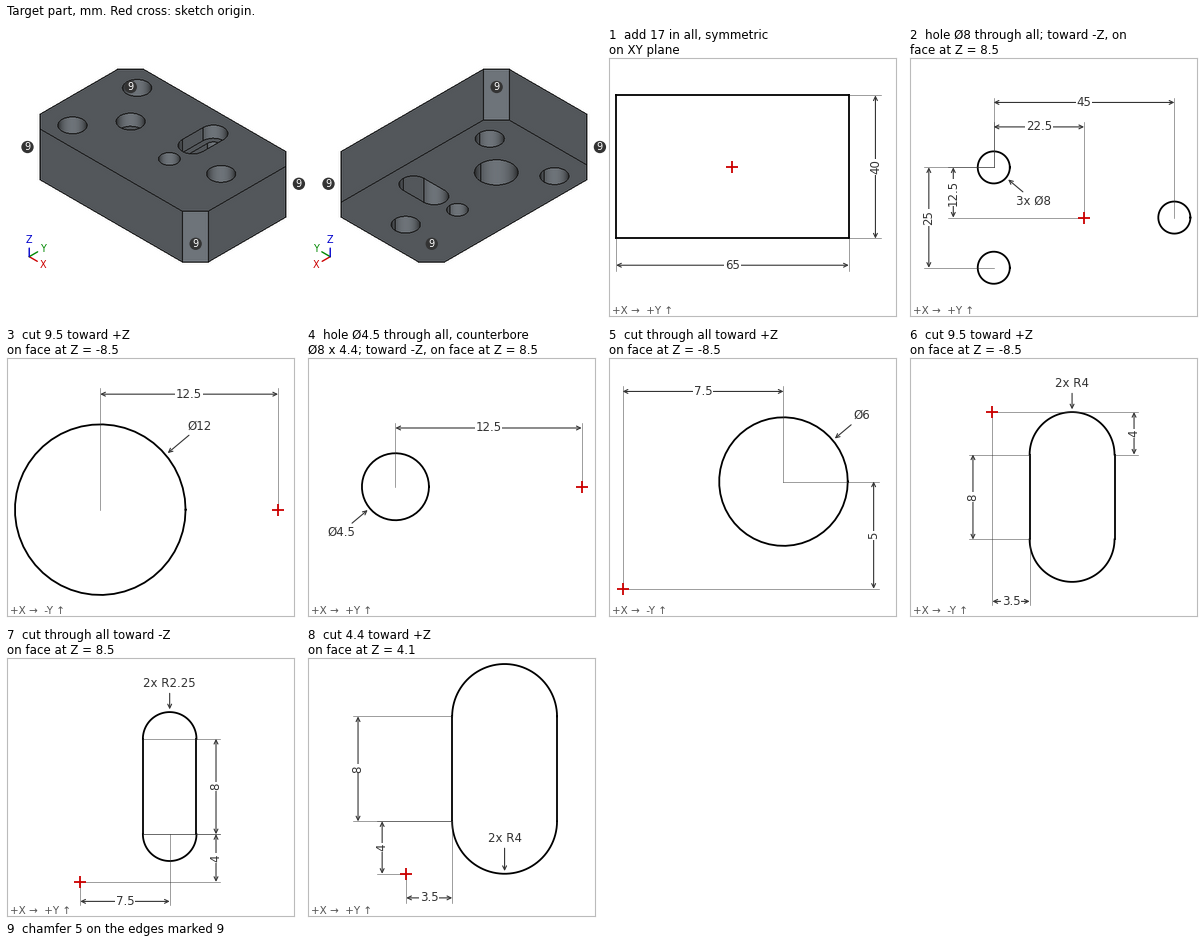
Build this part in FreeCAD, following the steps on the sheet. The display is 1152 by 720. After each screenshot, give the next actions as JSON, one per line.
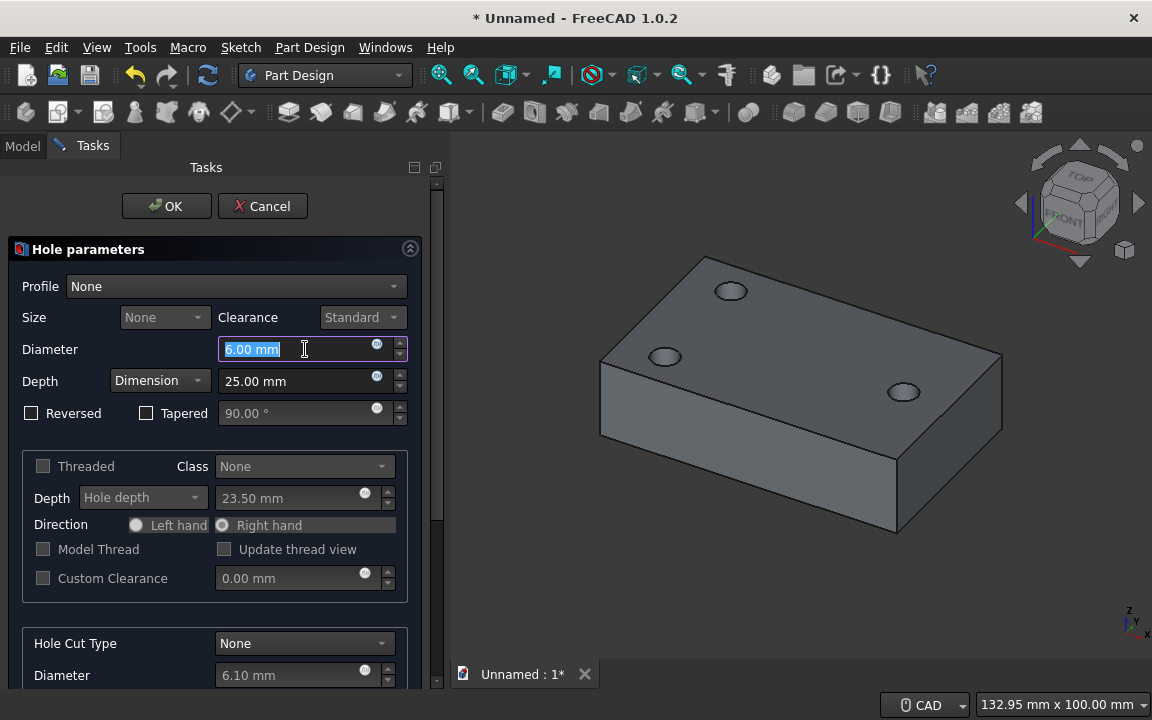
{"action": "type", "text": "8"}
{"action": "key", "text": "Tab"}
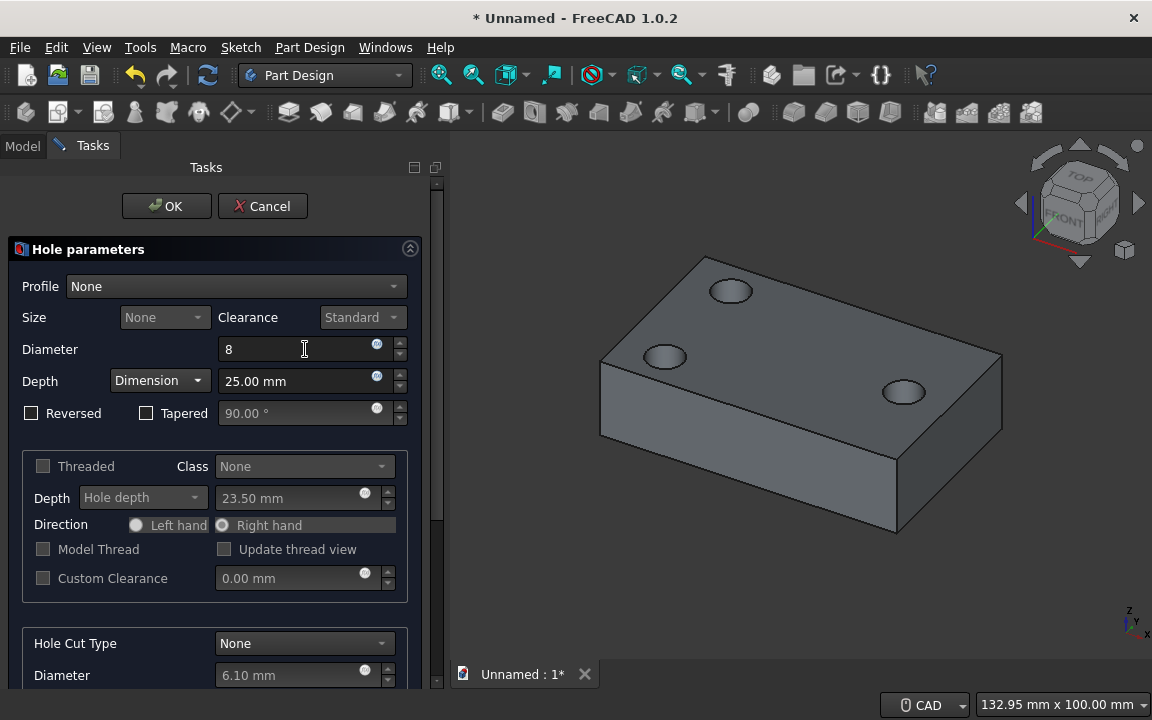
{"action": "left_click", "coordinate": [161, 380]}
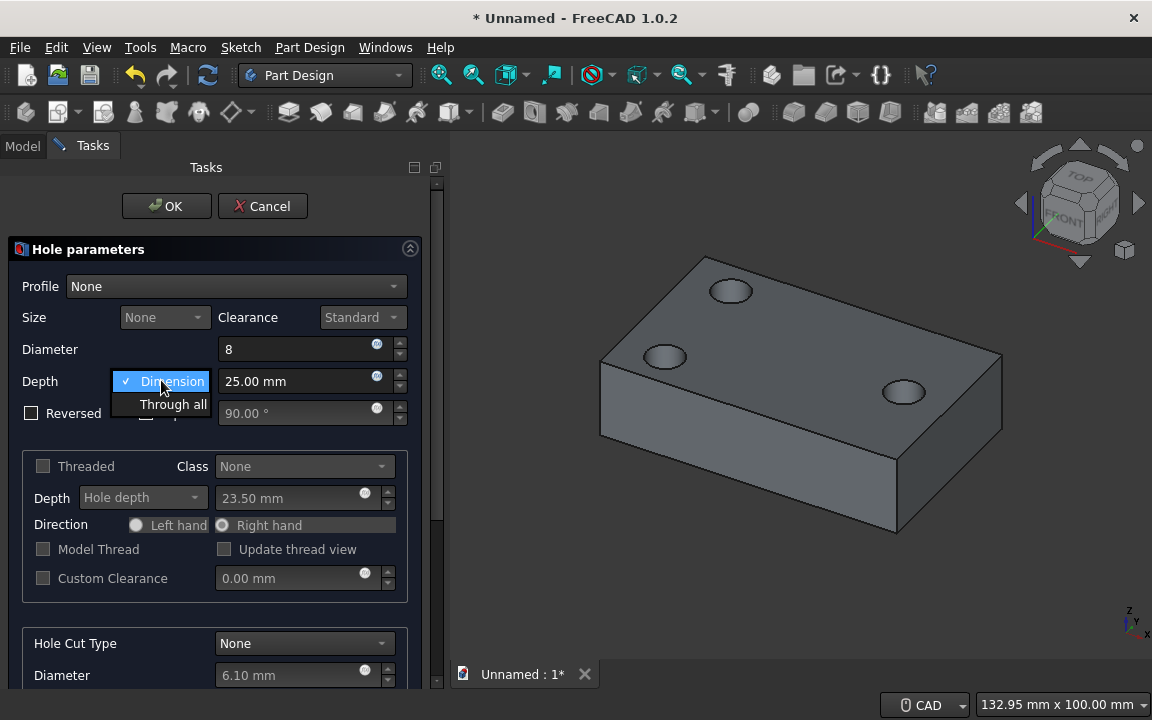
{"action": "left_click", "coordinate": [160, 404]}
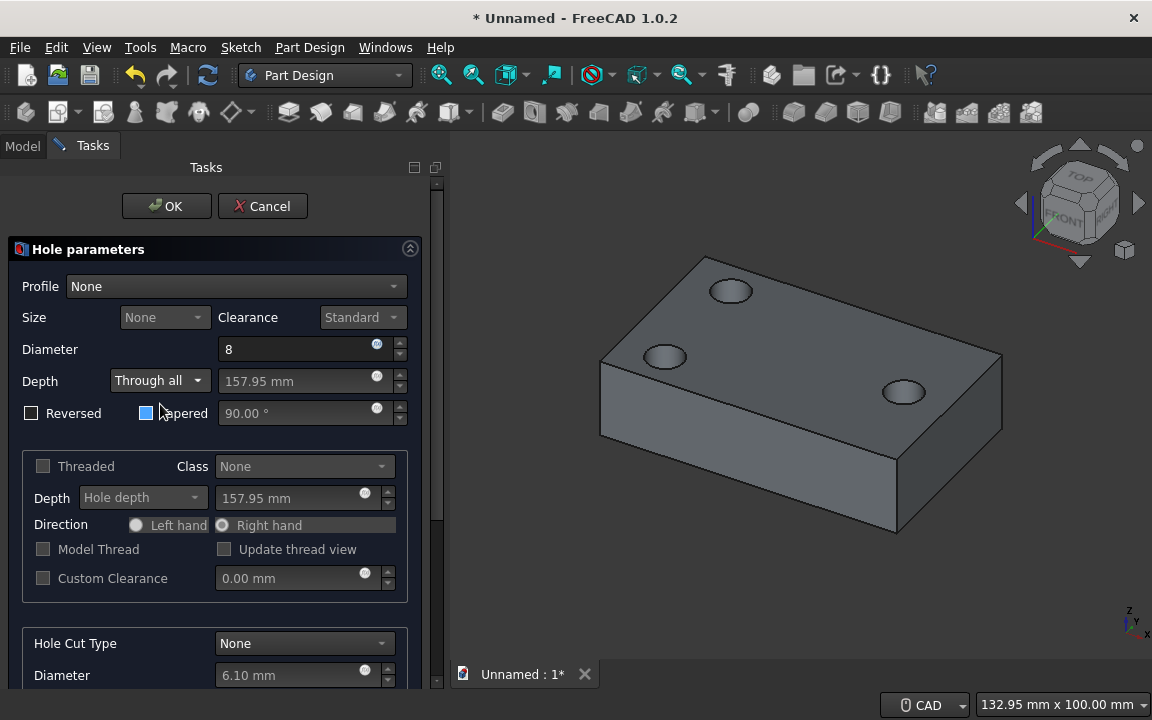
{"action": "left_click", "coordinate": [167, 206]}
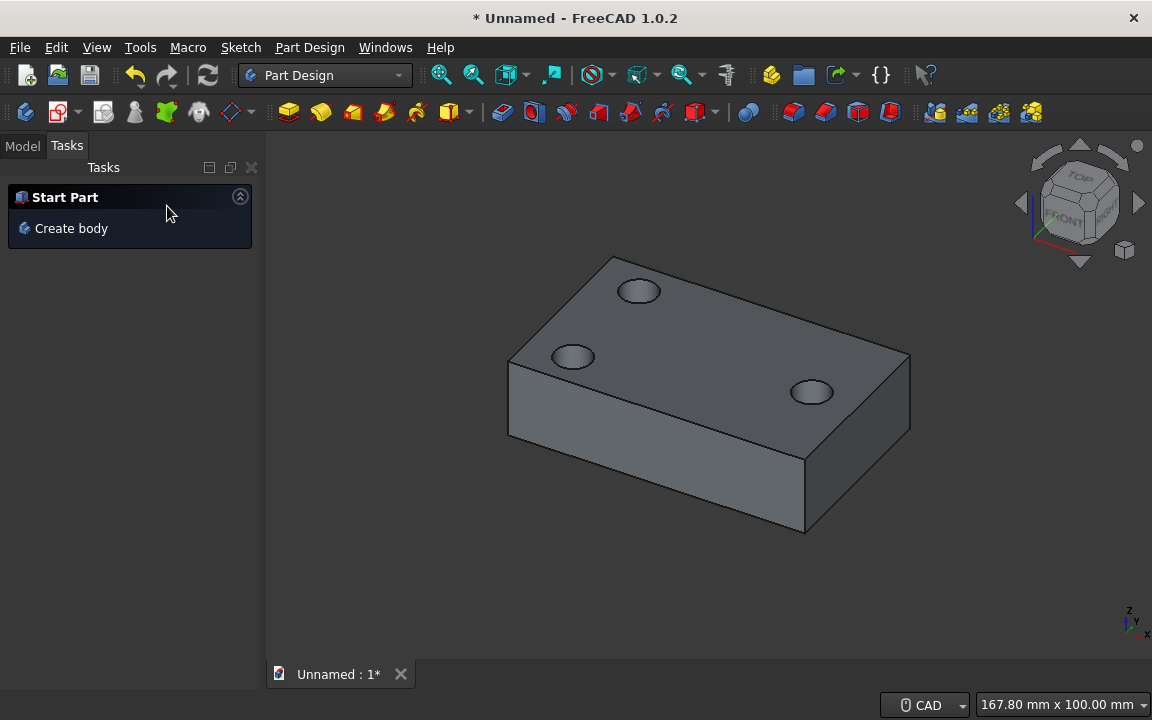
{"action": "key", "text": "5"}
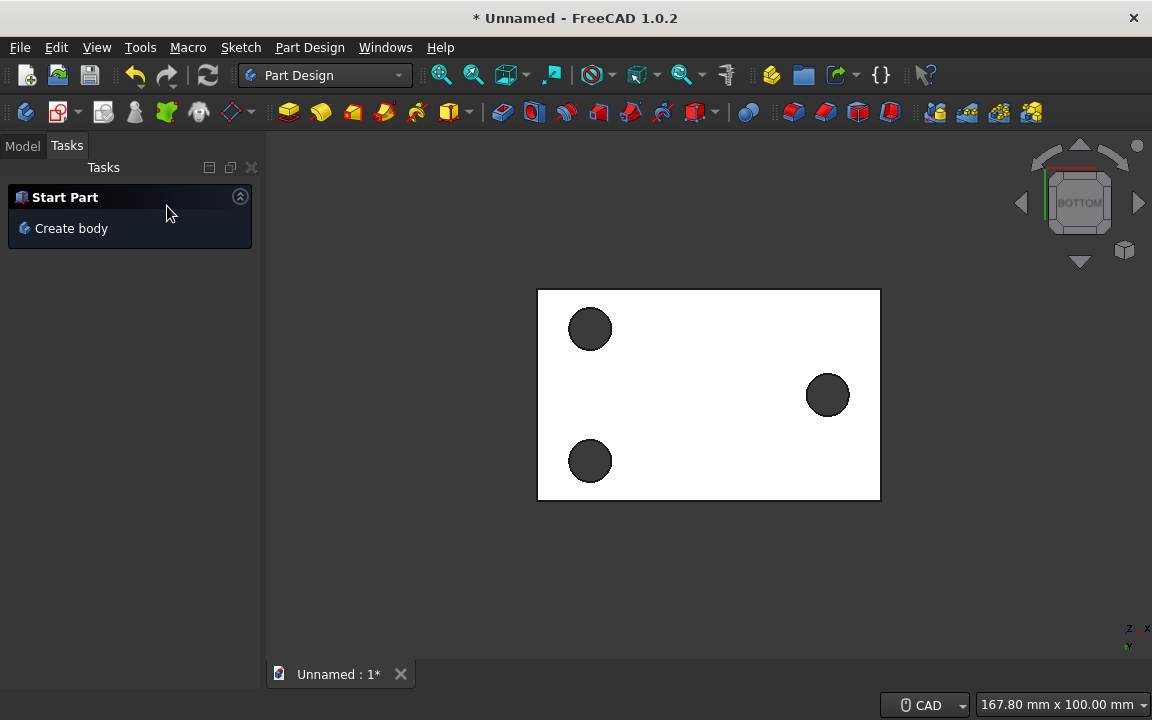
{"action": "left_click", "coordinate": [442, 76]}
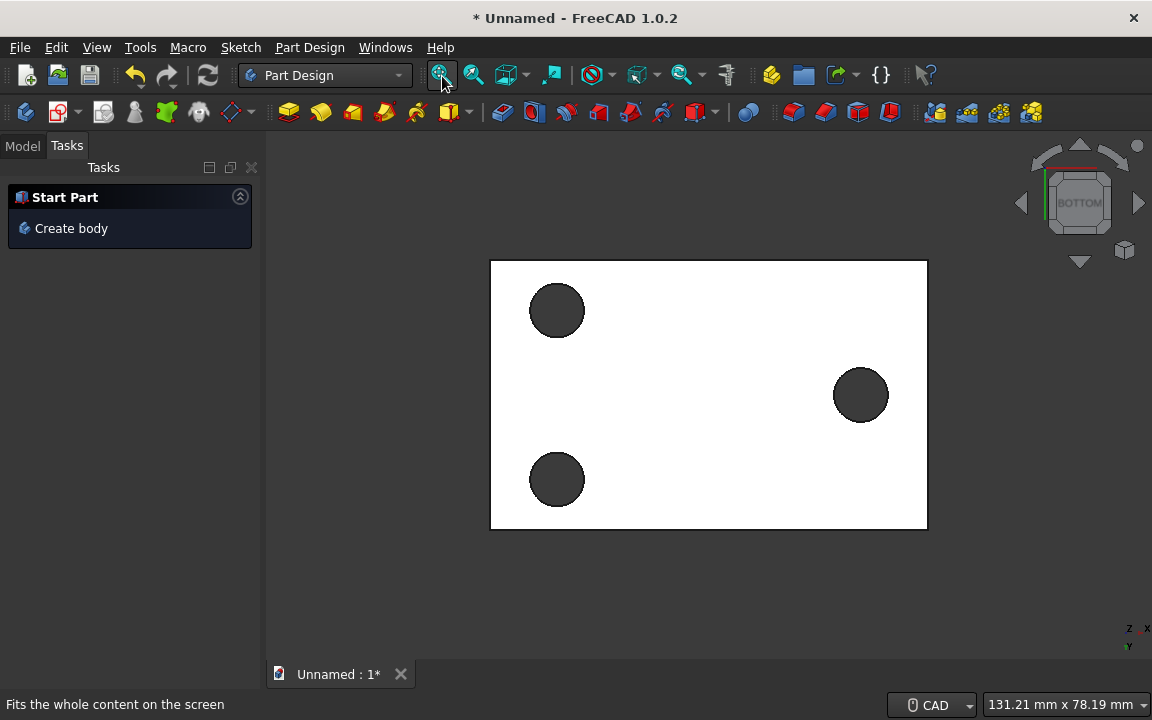
{"action": "left_click", "coordinate": [709, 394]}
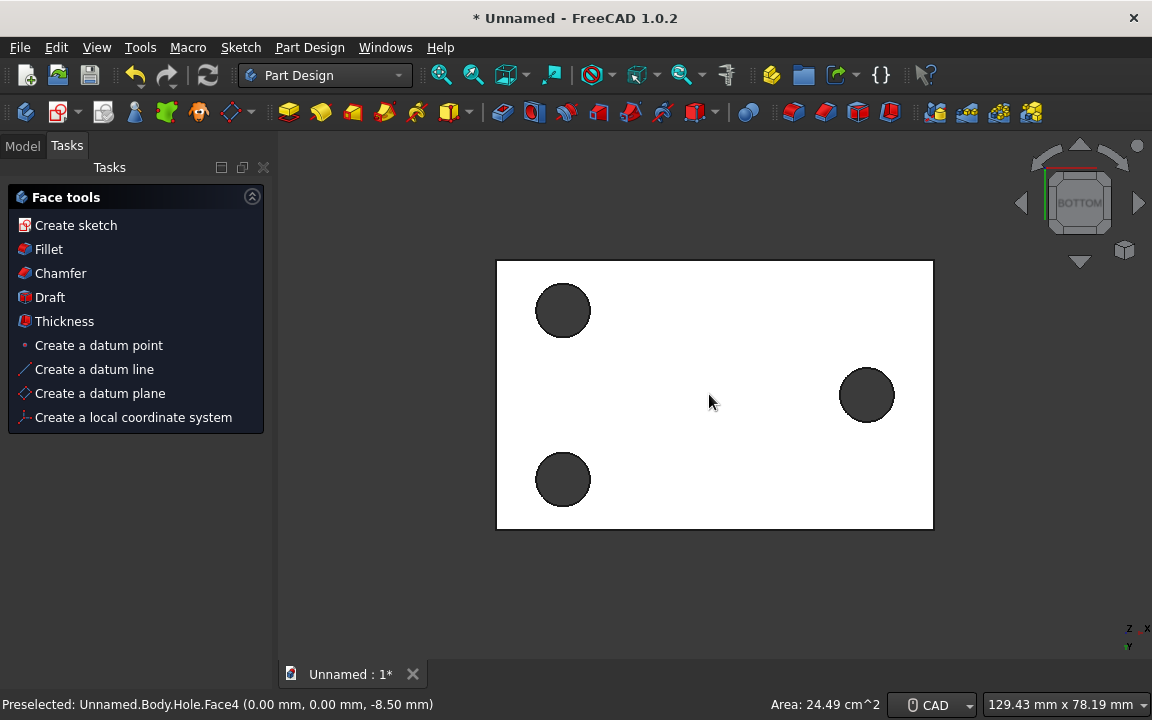
{"action": "left_click", "coordinate": [58, 112]}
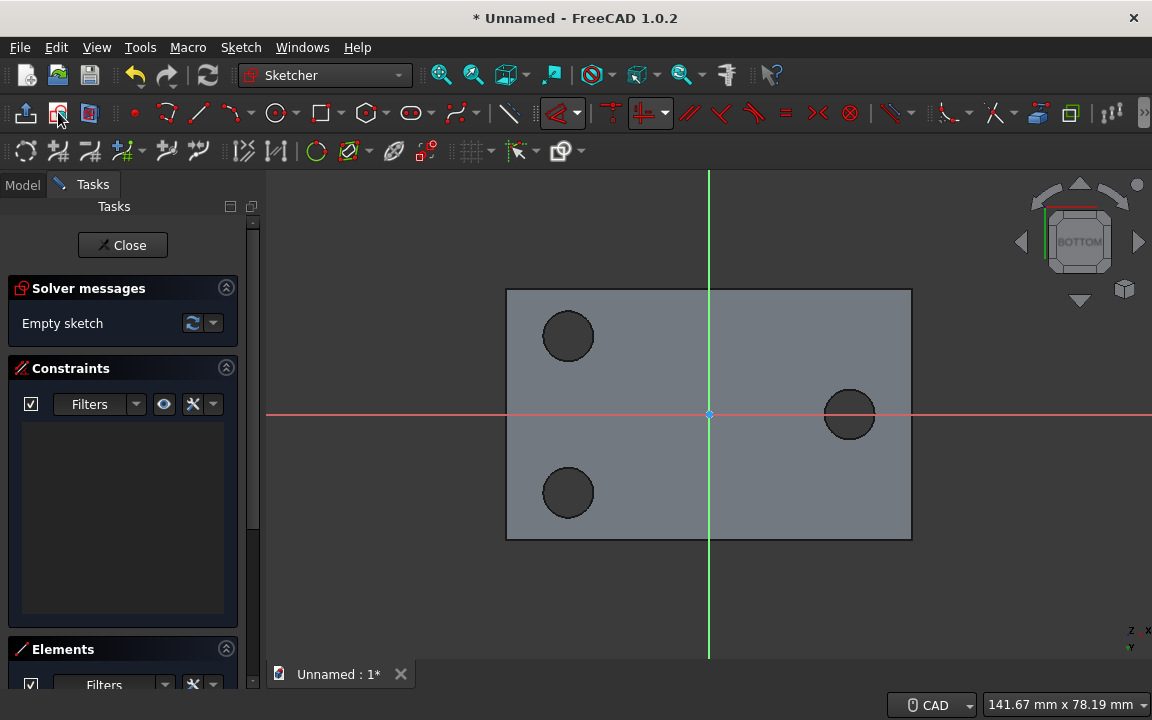
{"action": "scroll", "coordinate": [655, 415], "scroll_direction": "up", "scroll_amount": 7}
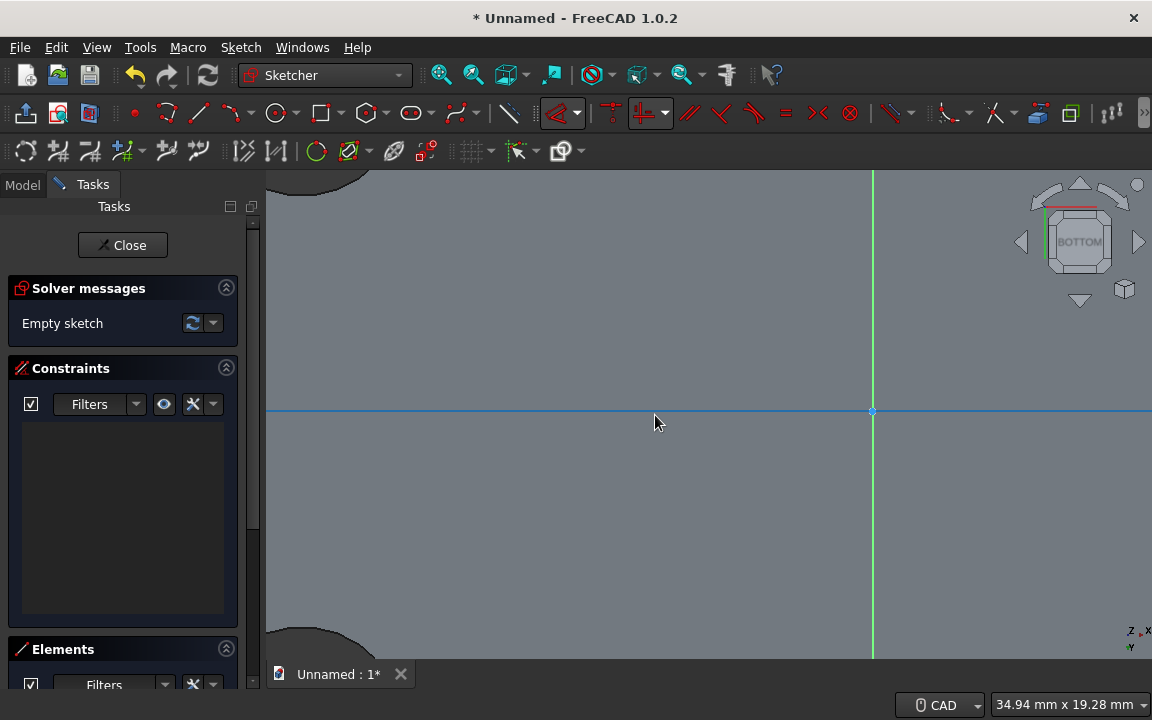
{"action": "key", "text": "g c"}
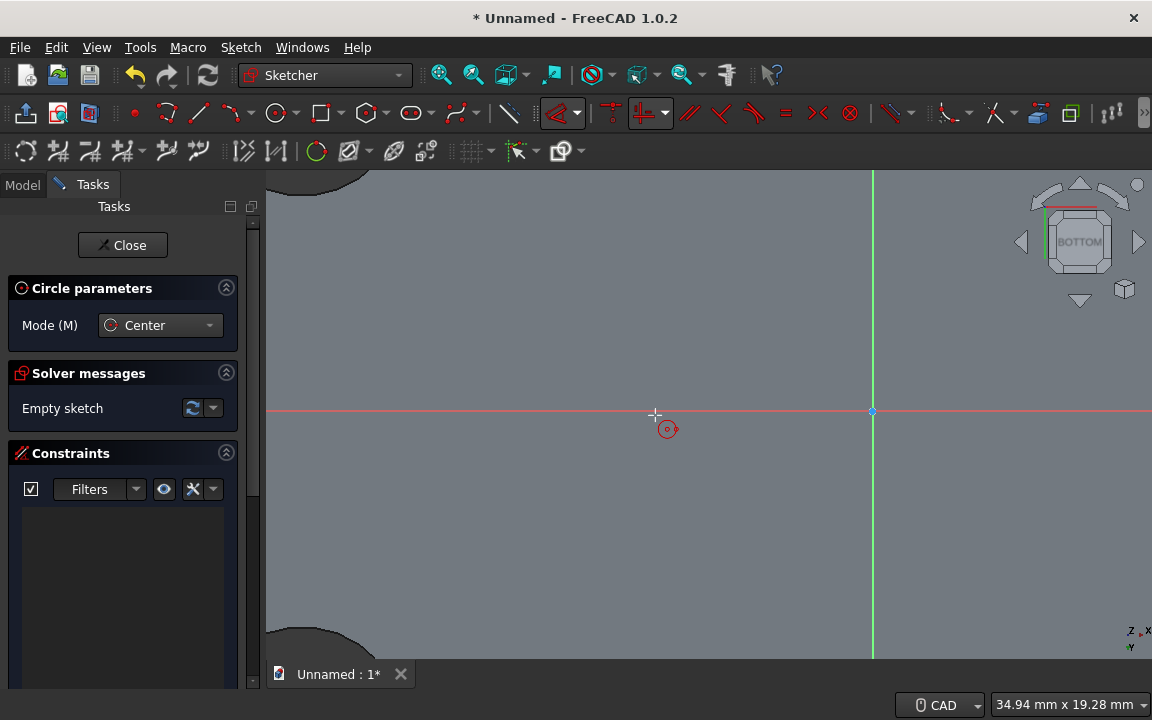
{"action": "left_click", "coordinate": [556, 411]}
{"action": "left_click", "coordinate": [663, 304]}
{"action": "key", "text": "Escape"}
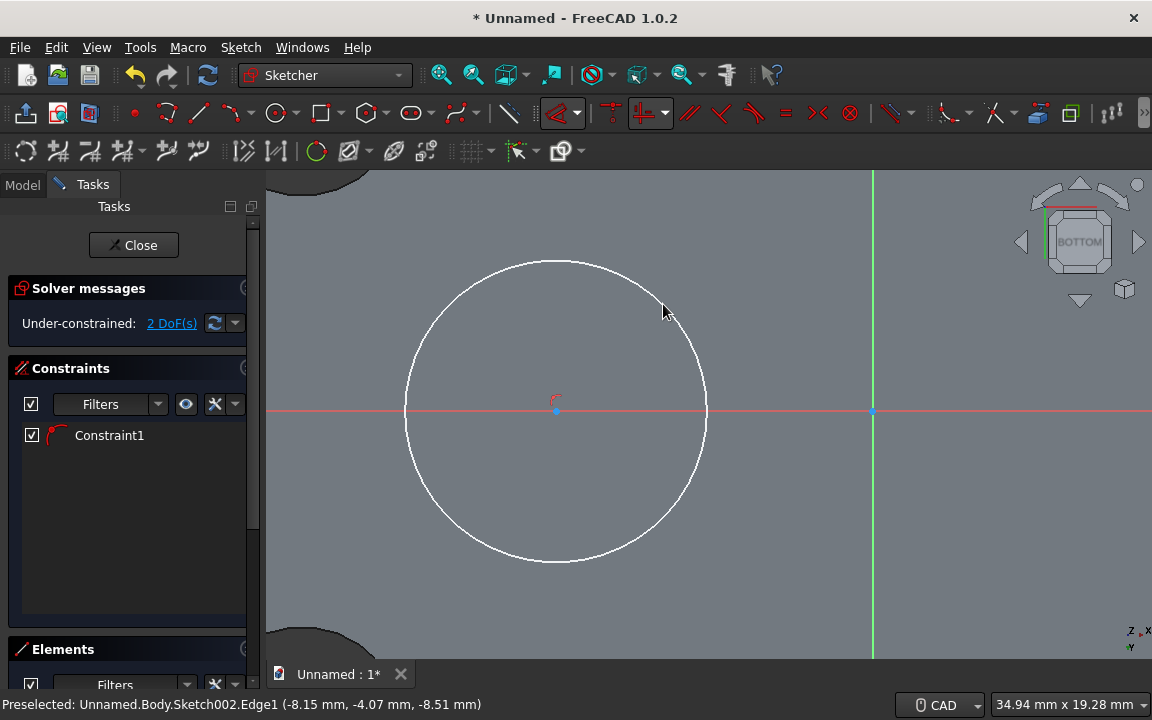
{"action": "left_click", "coordinate": [556, 114]}